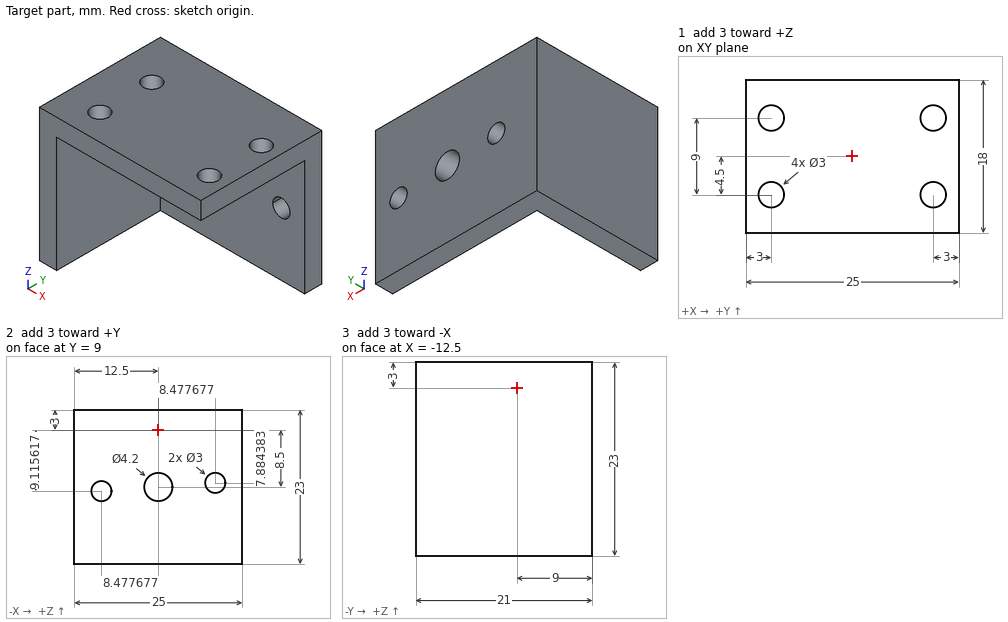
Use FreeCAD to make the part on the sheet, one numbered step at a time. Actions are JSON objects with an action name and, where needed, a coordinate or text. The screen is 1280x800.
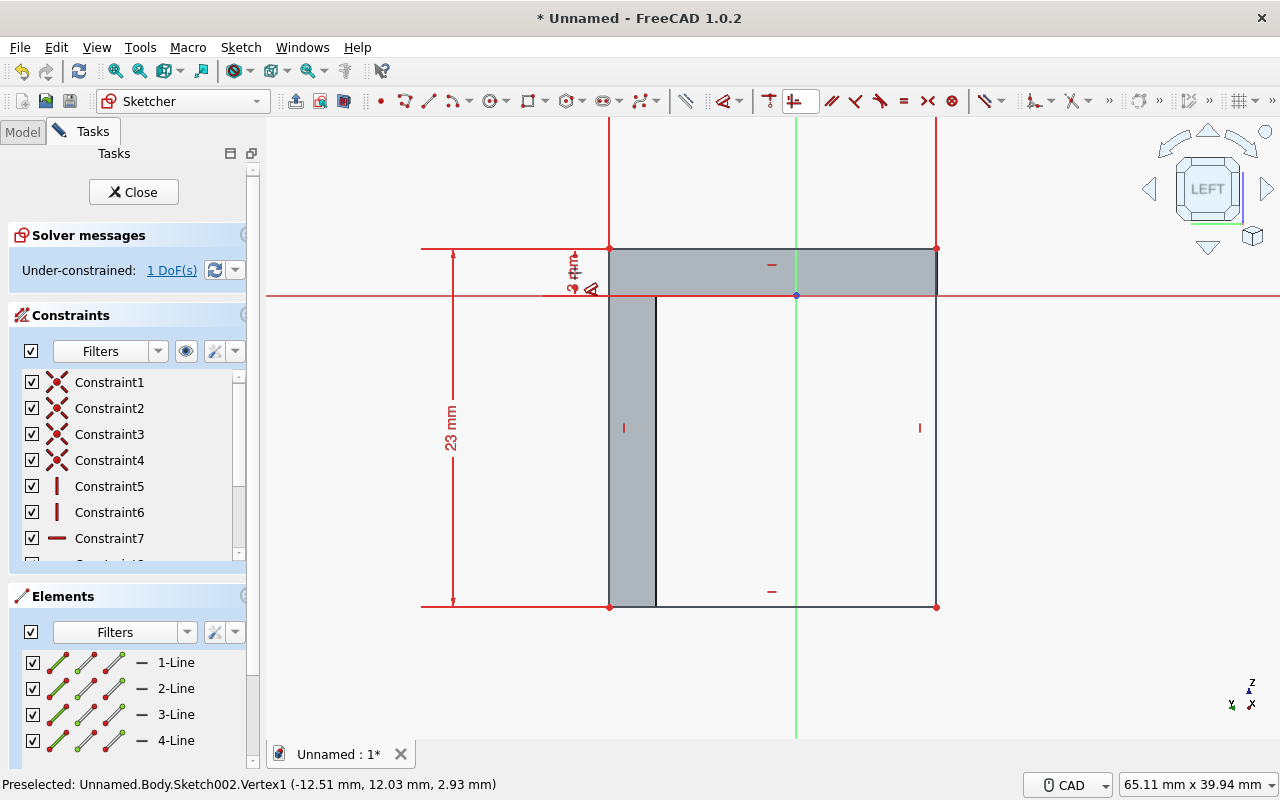
{"action": "left_click", "coordinate": [936, 607]}
{"action": "left_click", "coordinate": [866, 641]}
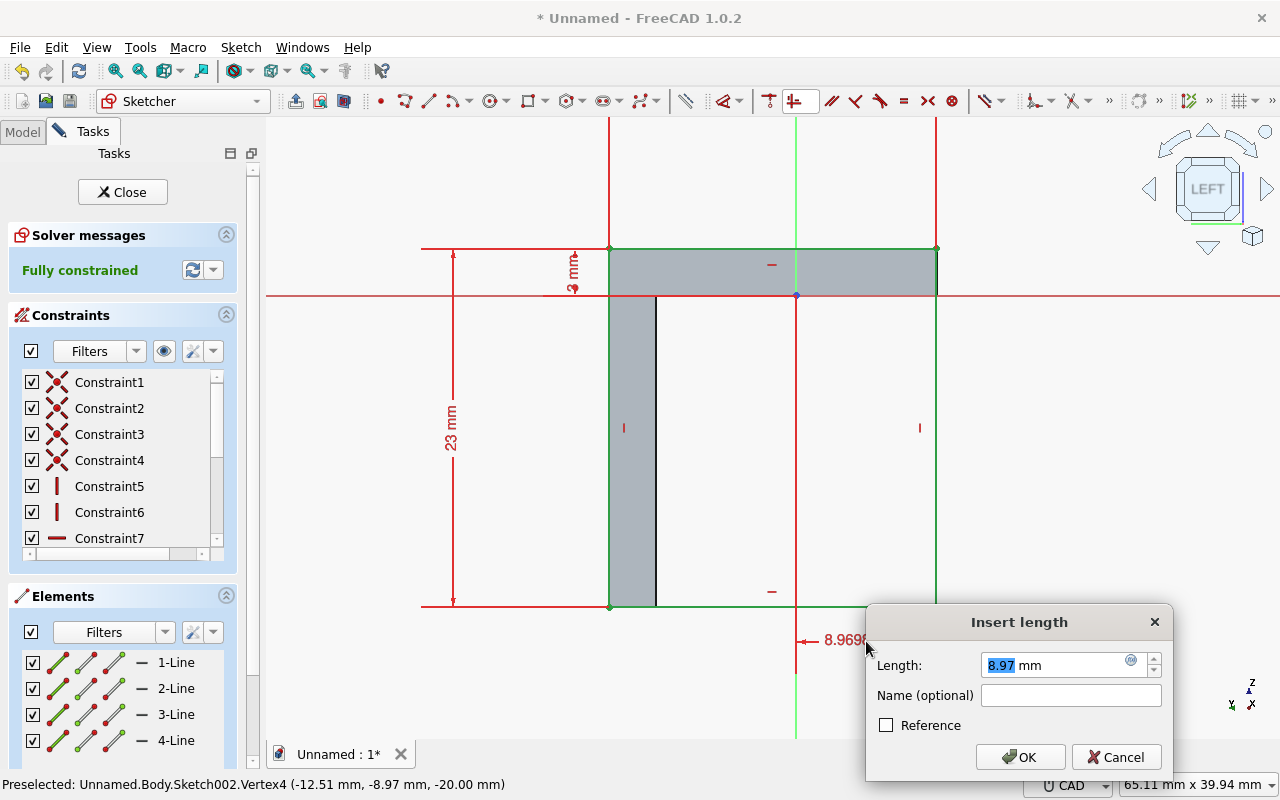
{"action": "type", "text": "9"}
{"action": "key", "text": "Return"}
{"action": "key", "text": "Escape"}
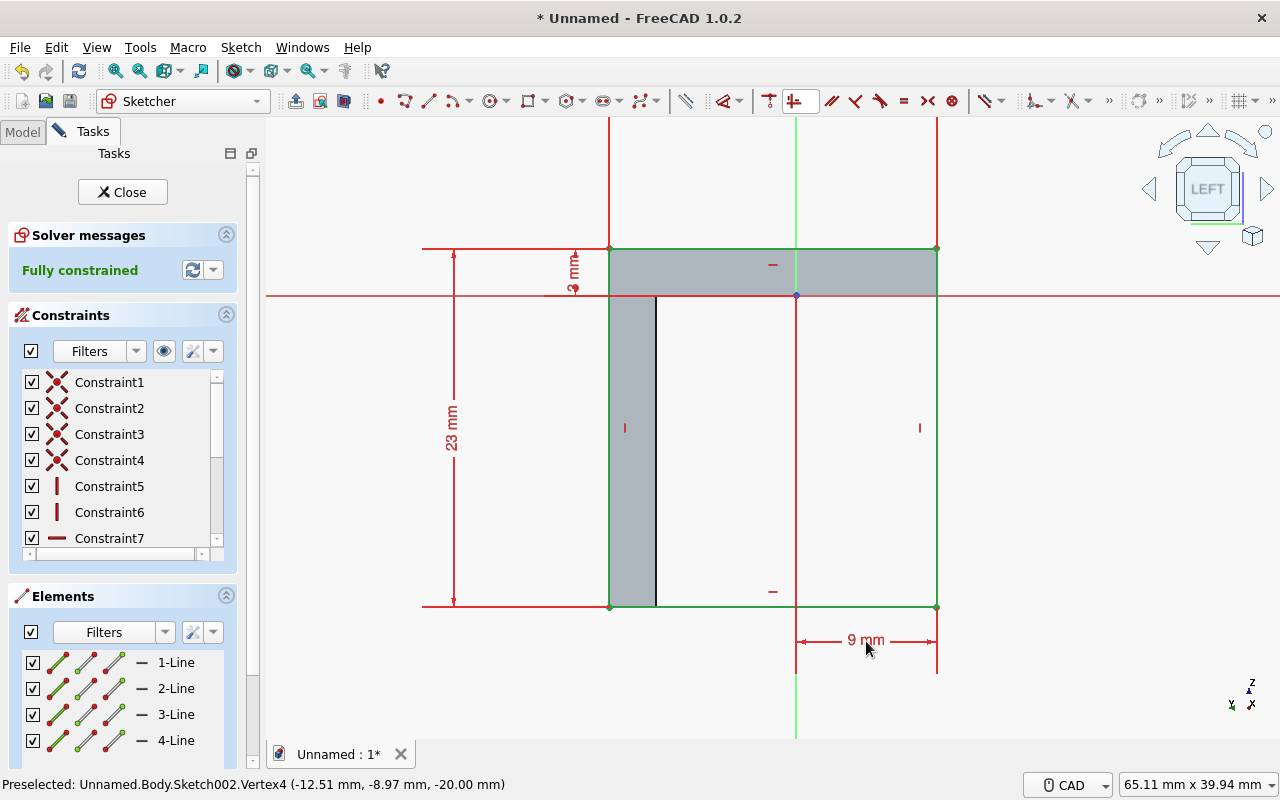
{"action": "left_click", "coordinate": [123, 192]}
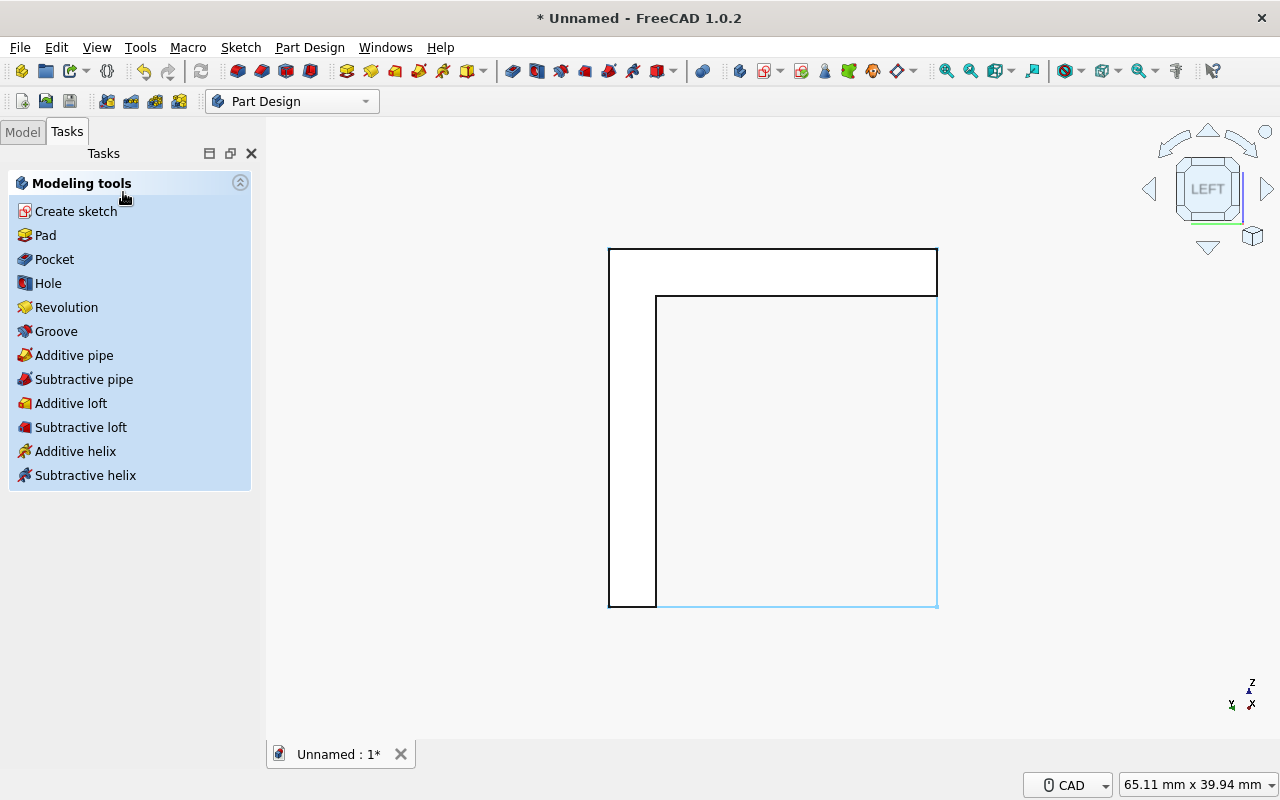
{"action": "left_click", "coordinate": [348, 72]}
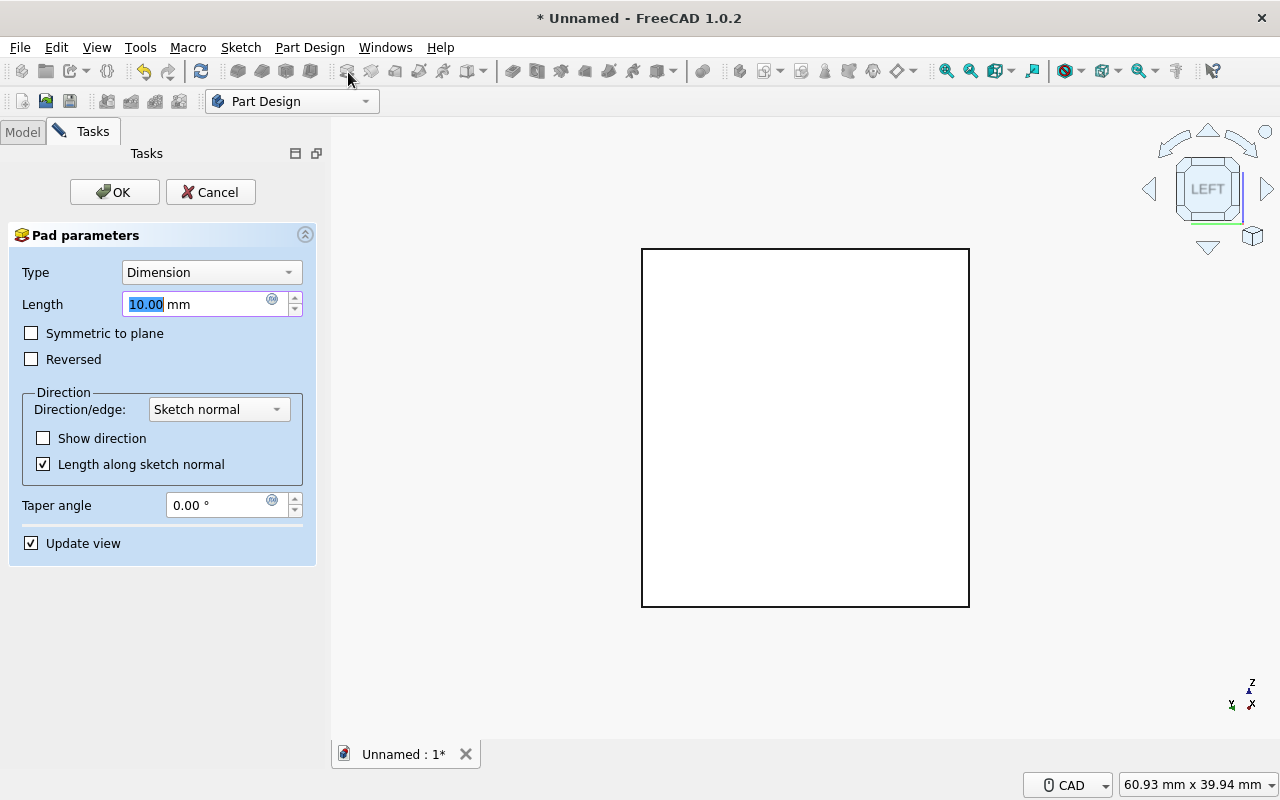
{"action": "type", "text": "3"}
{"action": "key", "text": "Tab"}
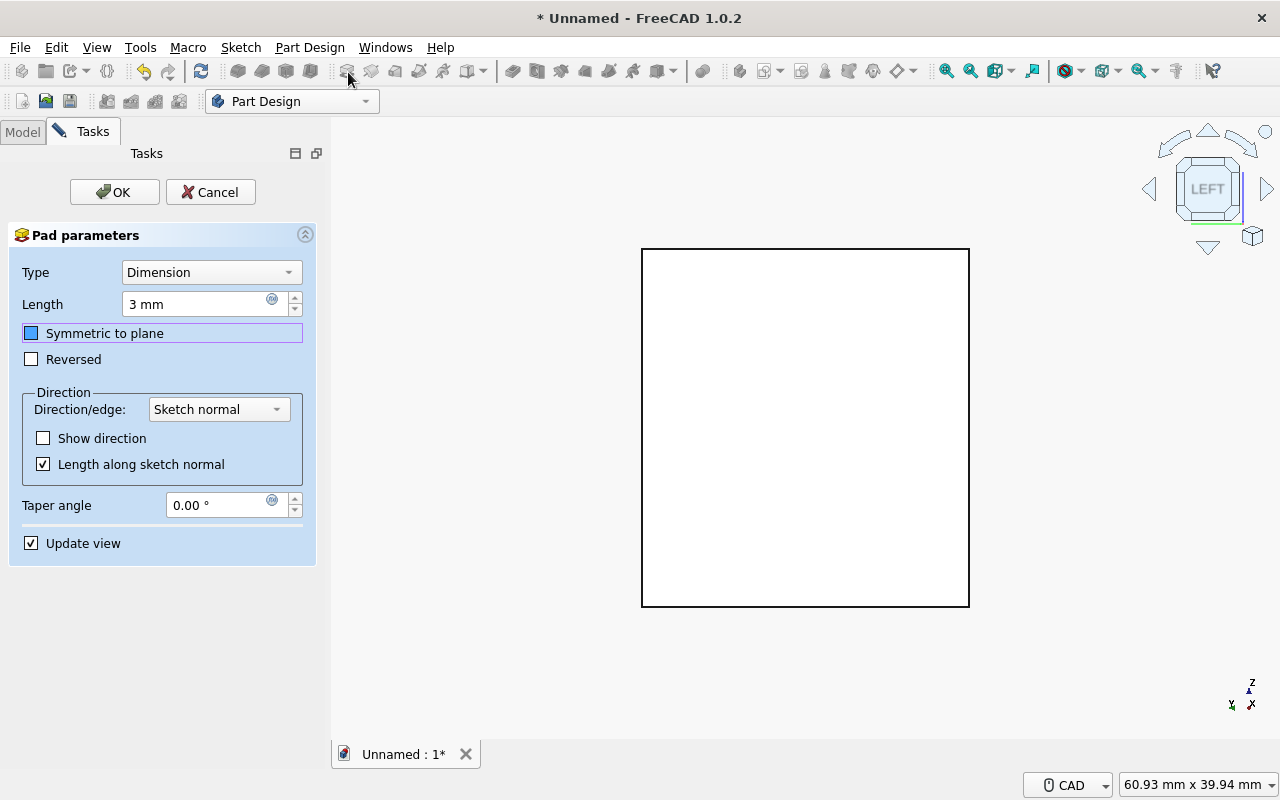
{"action": "left_click", "coordinate": [115, 192]}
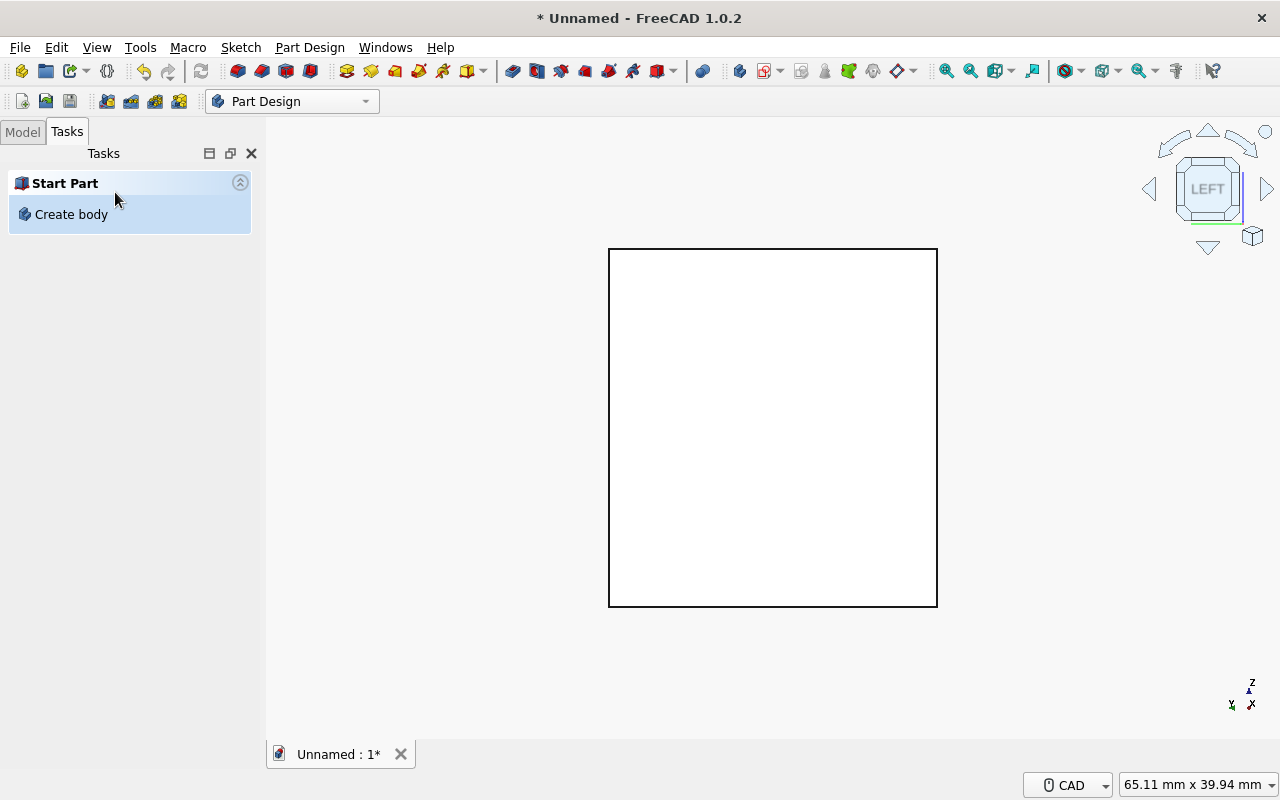
{"action": "key", "text": "0"}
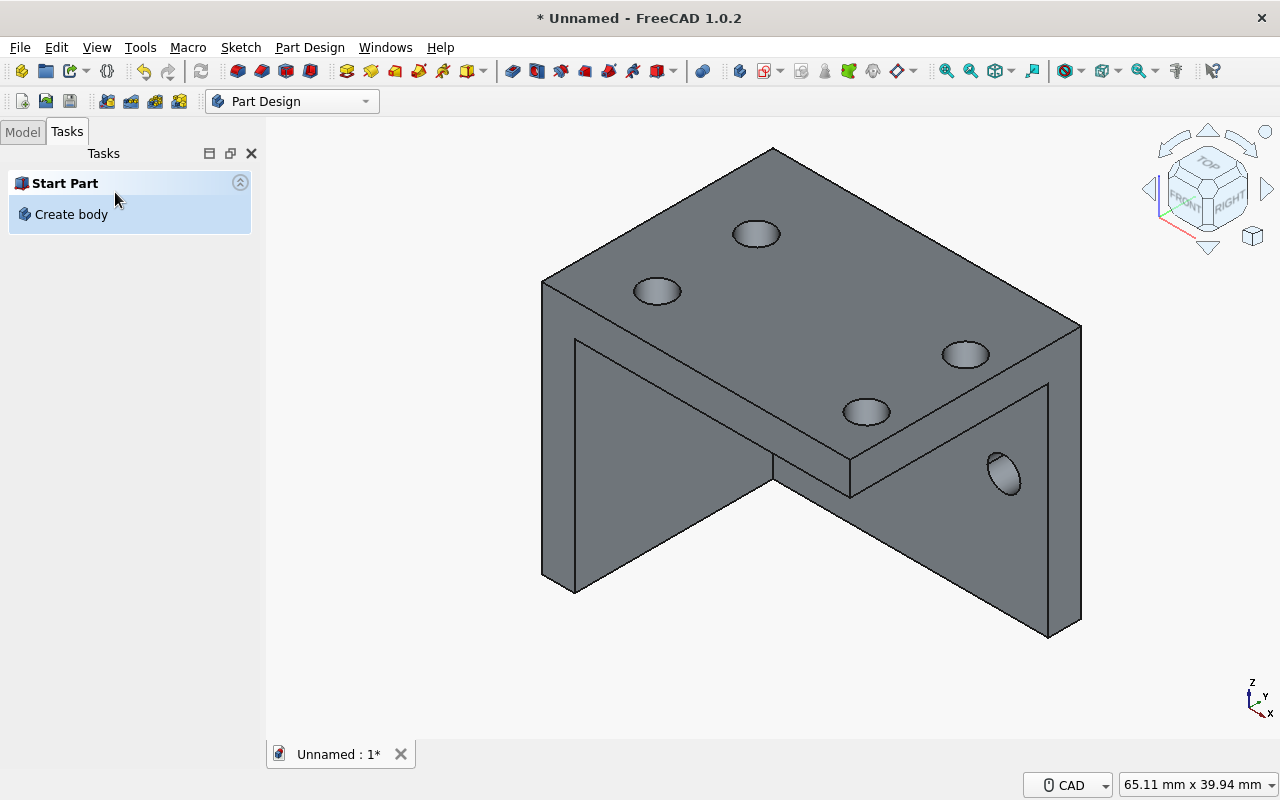
{"action": "key", "text": "v f"}